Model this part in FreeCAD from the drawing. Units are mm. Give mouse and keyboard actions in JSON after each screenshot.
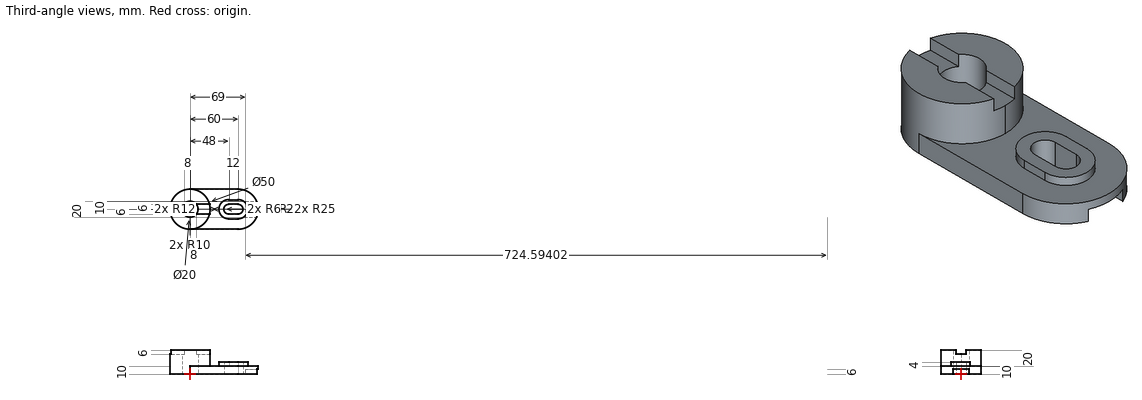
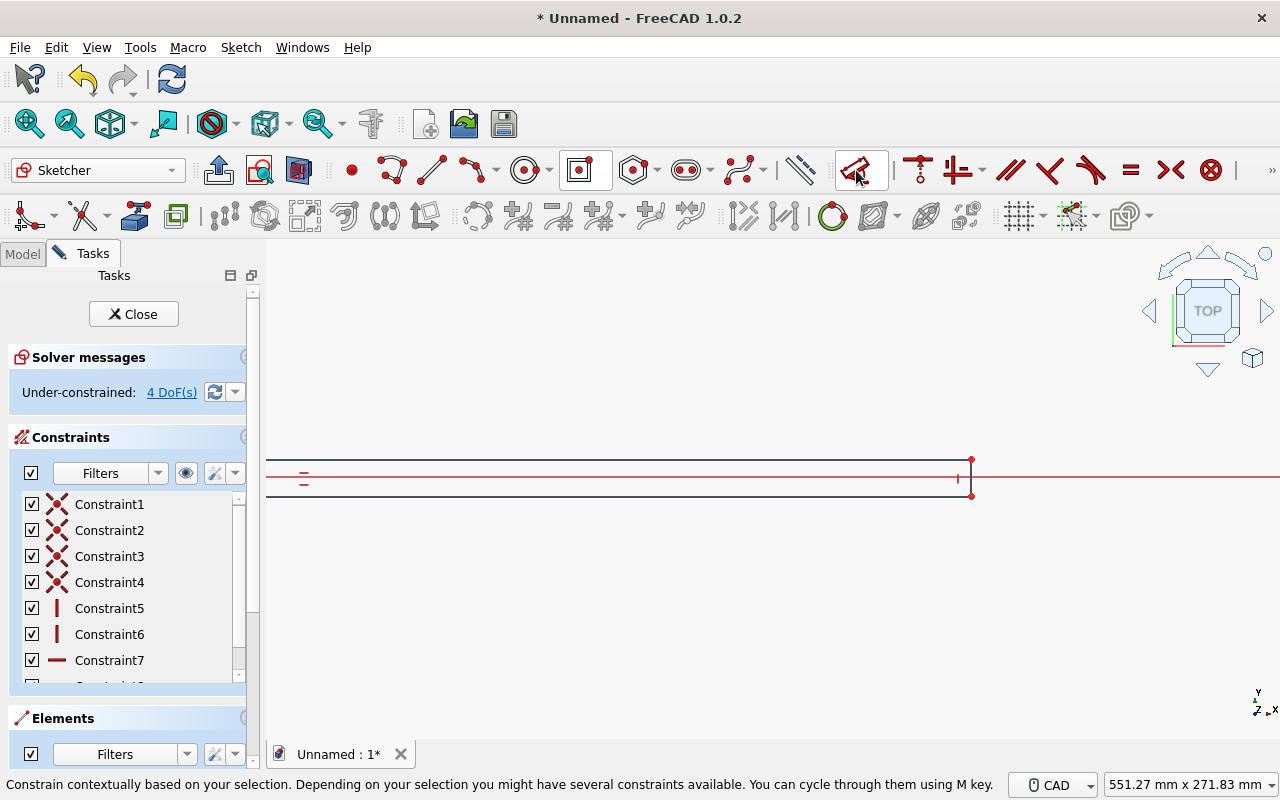
{"action": "scroll", "coordinate": [974, 496], "scroll_direction": "down", "scroll_amount": 5}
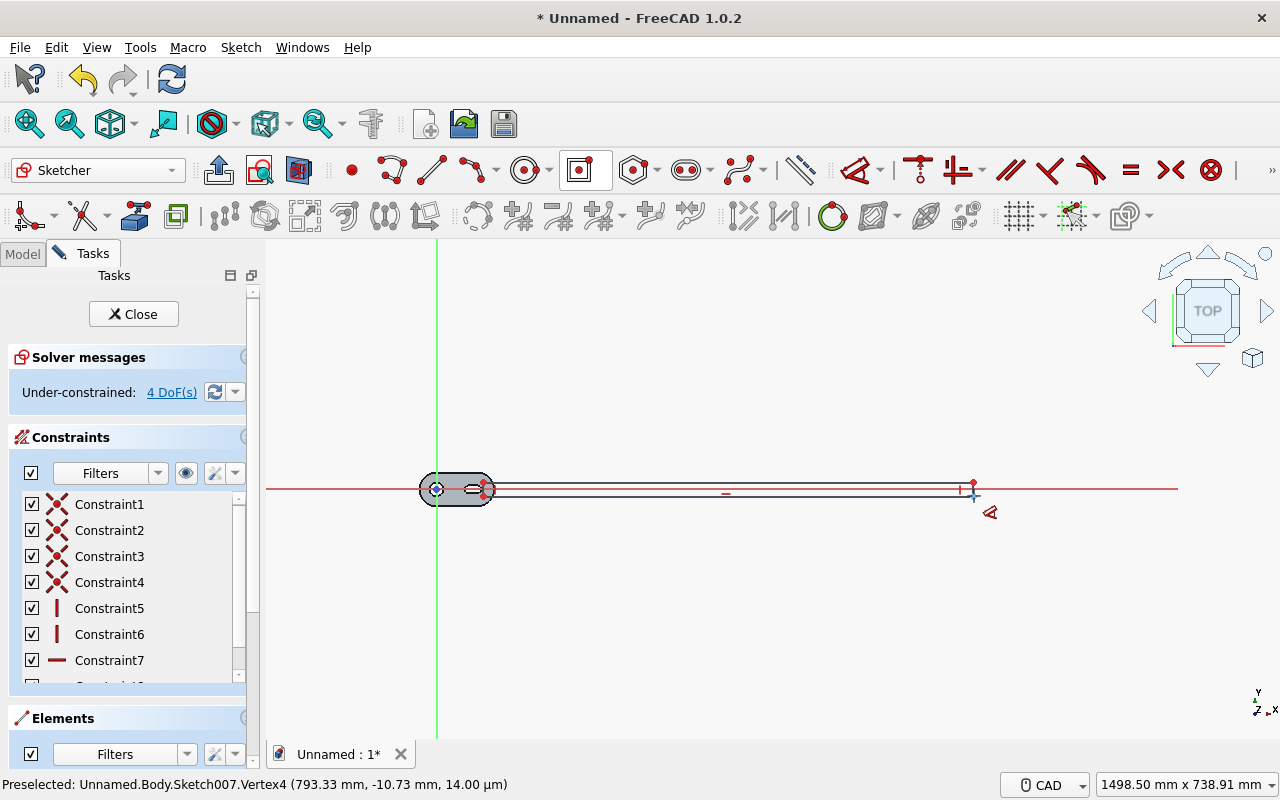
{"action": "scroll", "coordinate": [483, 488], "scroll_direction": "up", "scroll_amount": 6}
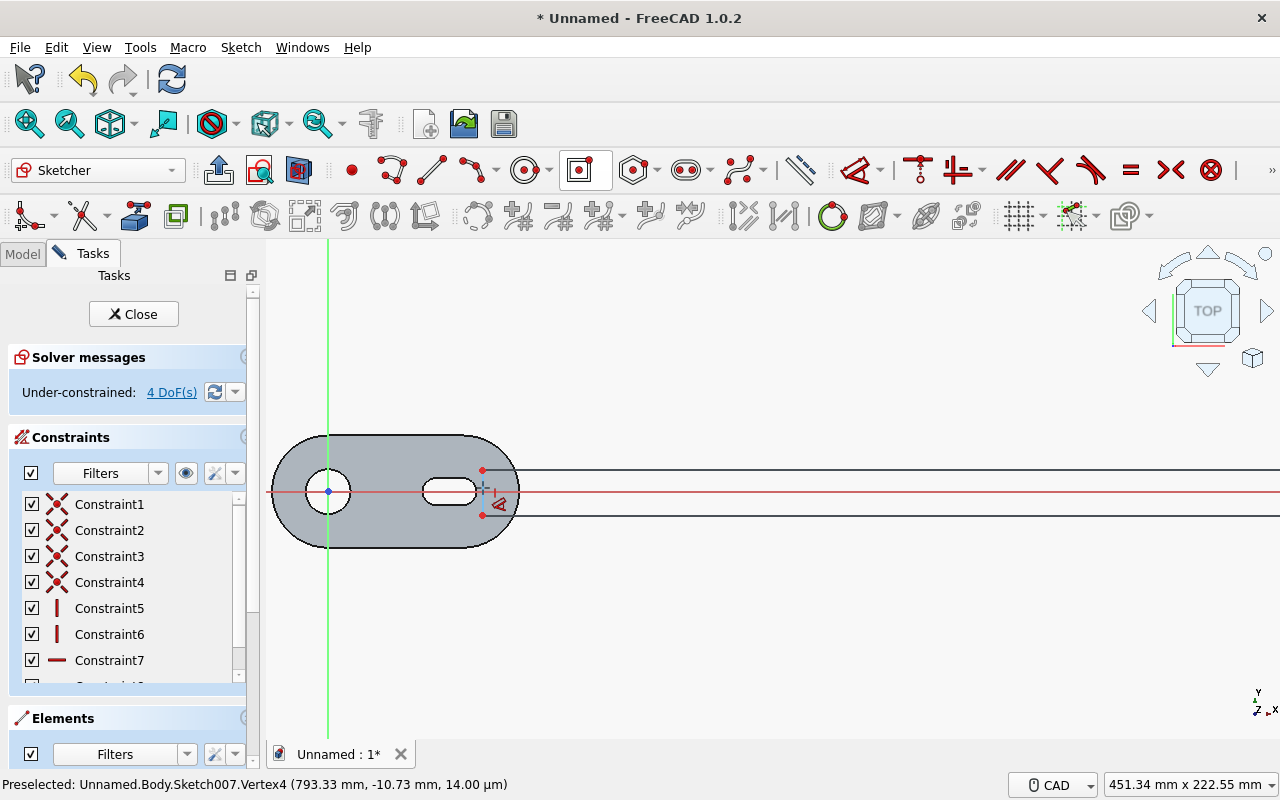
{"action": "left_click", "coordinate": [483, 488]}
{"action": "left_click", "coordinate": [449, 477]}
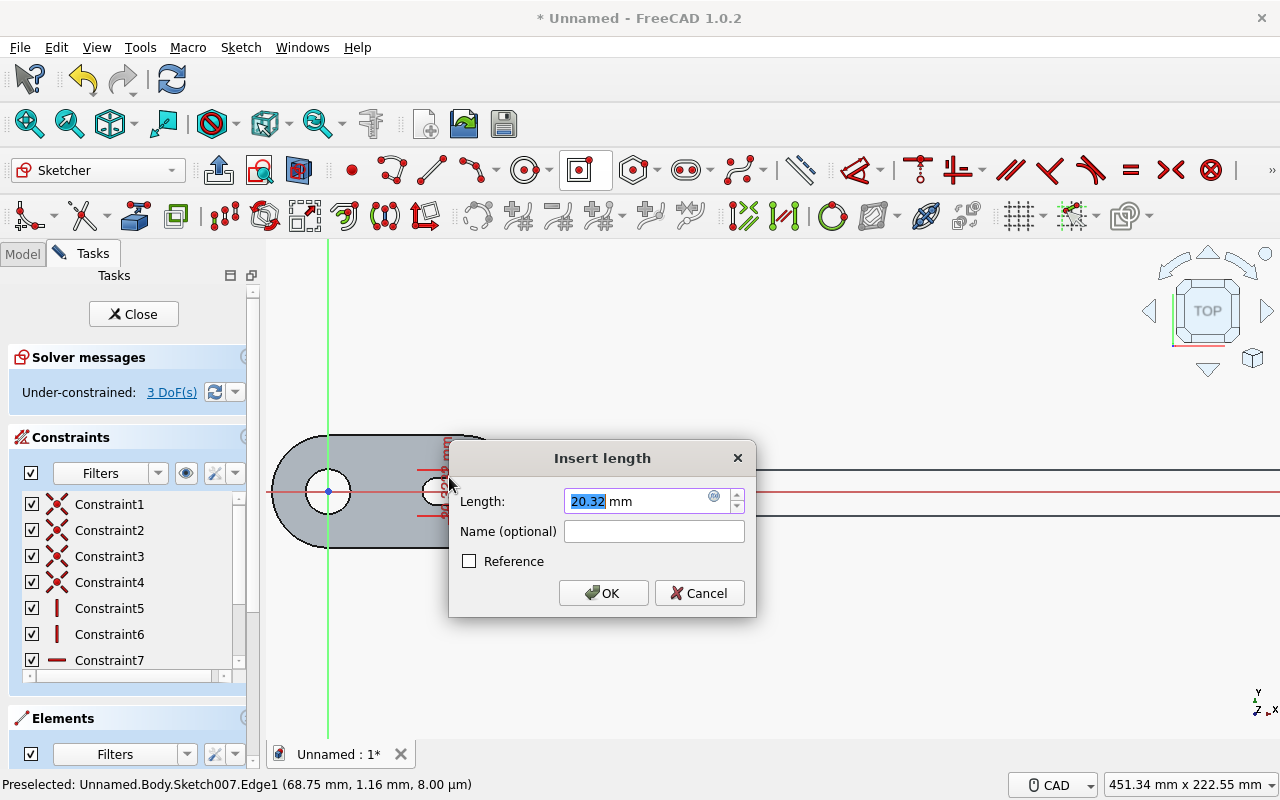
{"action": "type", "text": "20"}
{"action": "key", "text": "Return"}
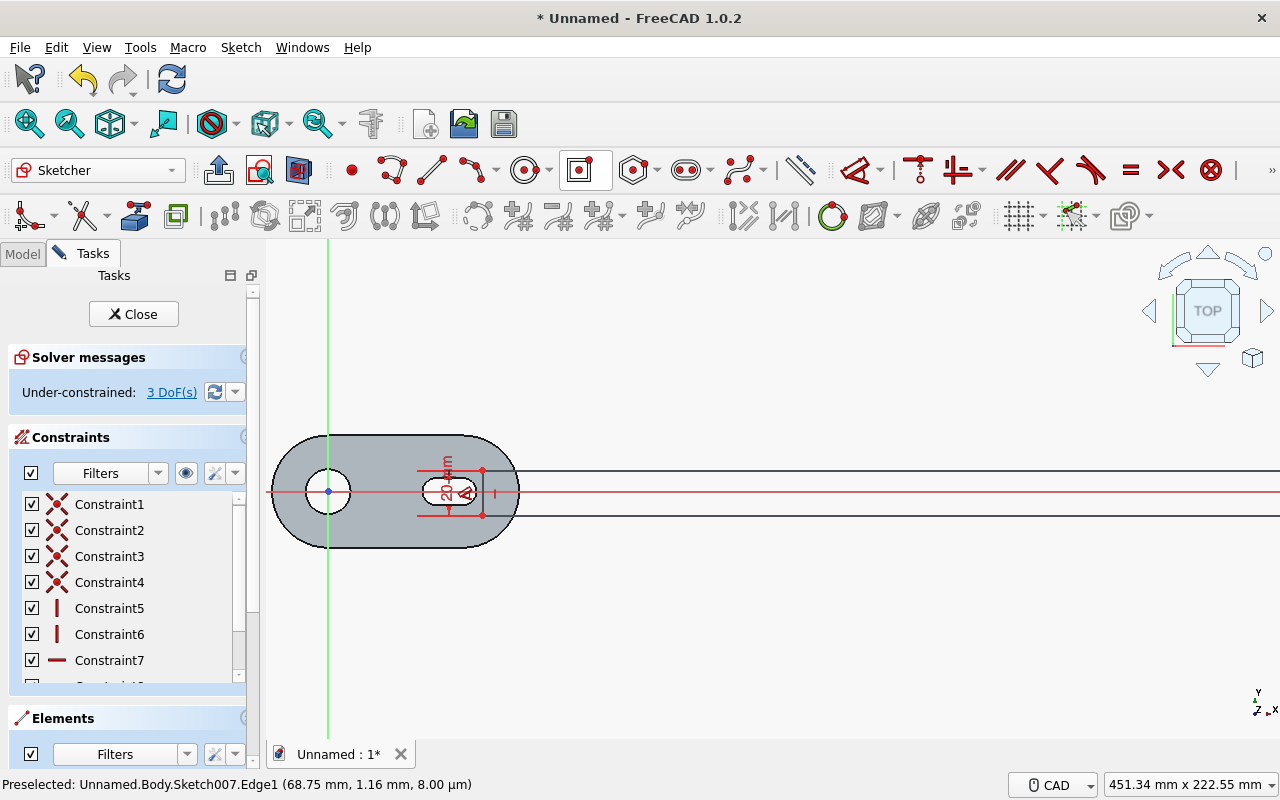
{"action": "left_click", "coordinate": [483, 471]}
{"action": "left_click", "coordinate": [405, 437]}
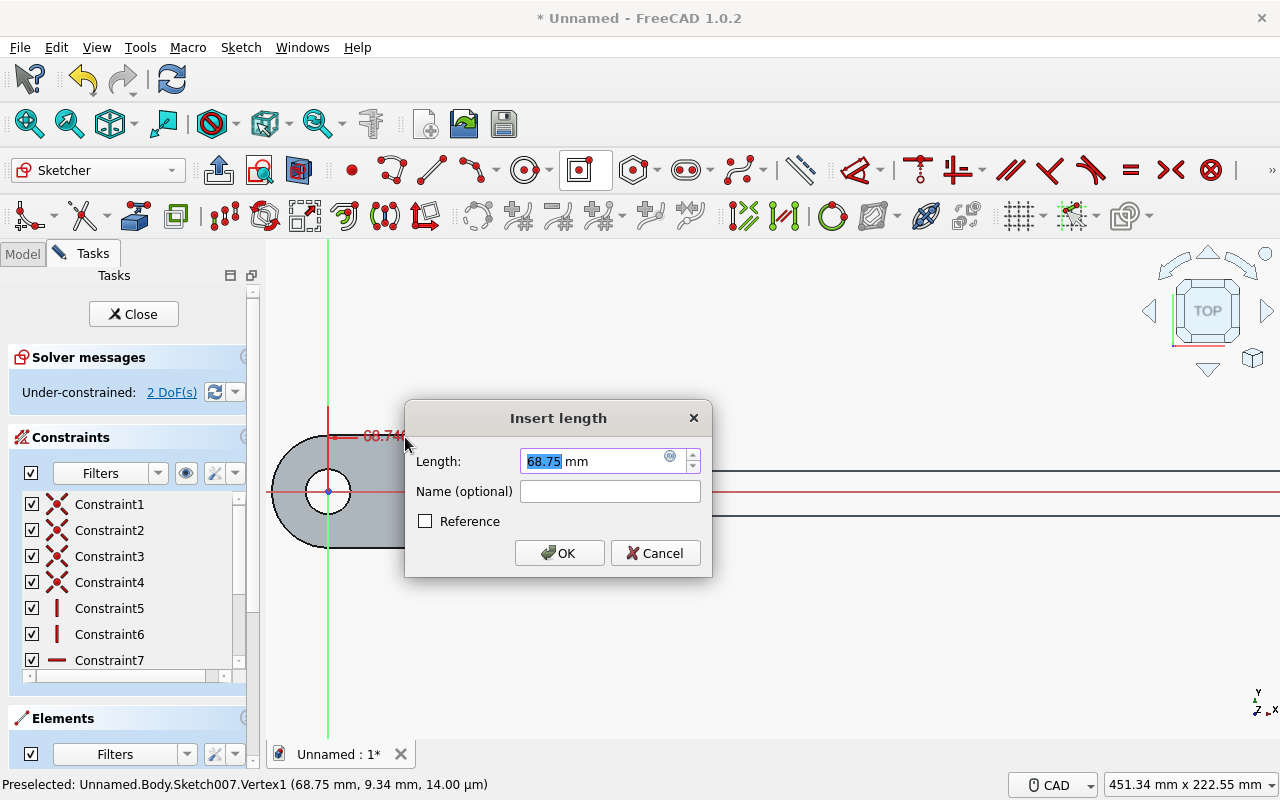
{"action": "type", "text": "69"}
{"action": "key", "text": "Return"}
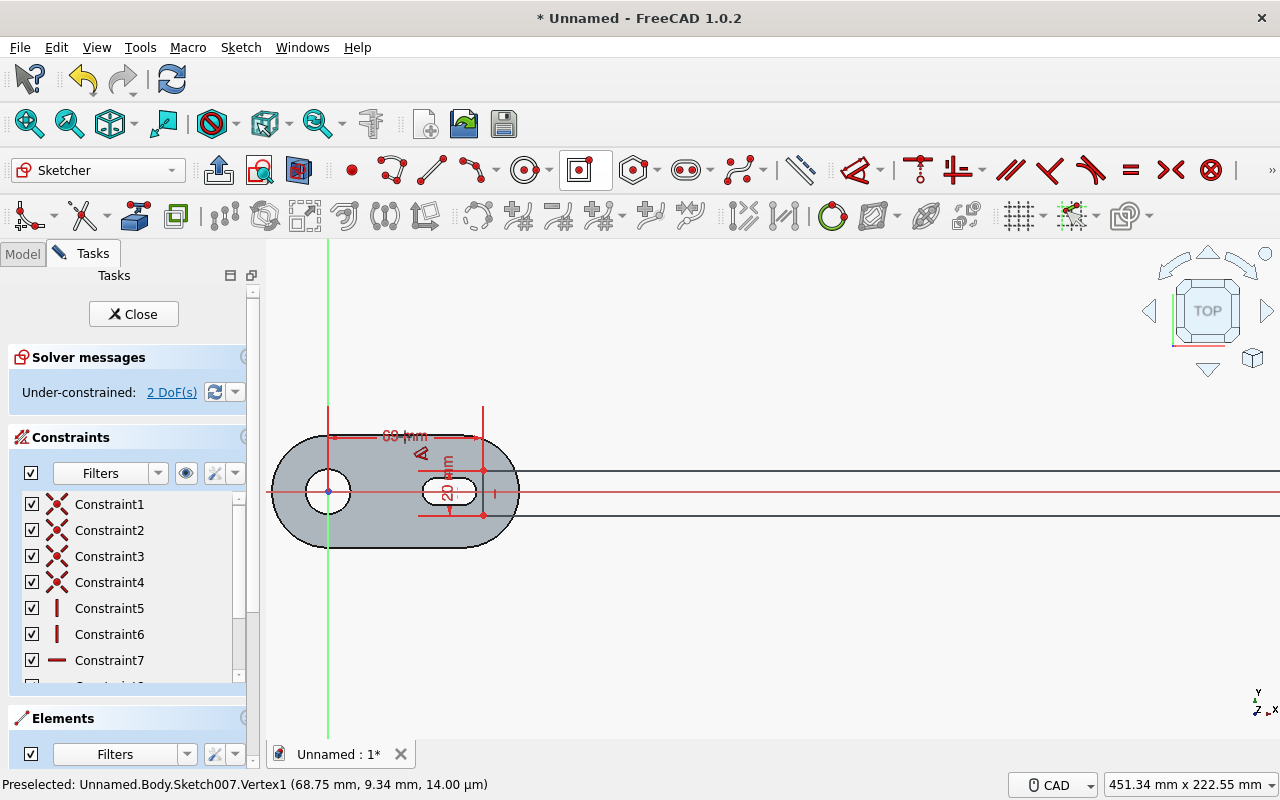
{"action": "scroll", "coordinate": [483, 471], "scroll_direction": "up", "scroll_amount": 3}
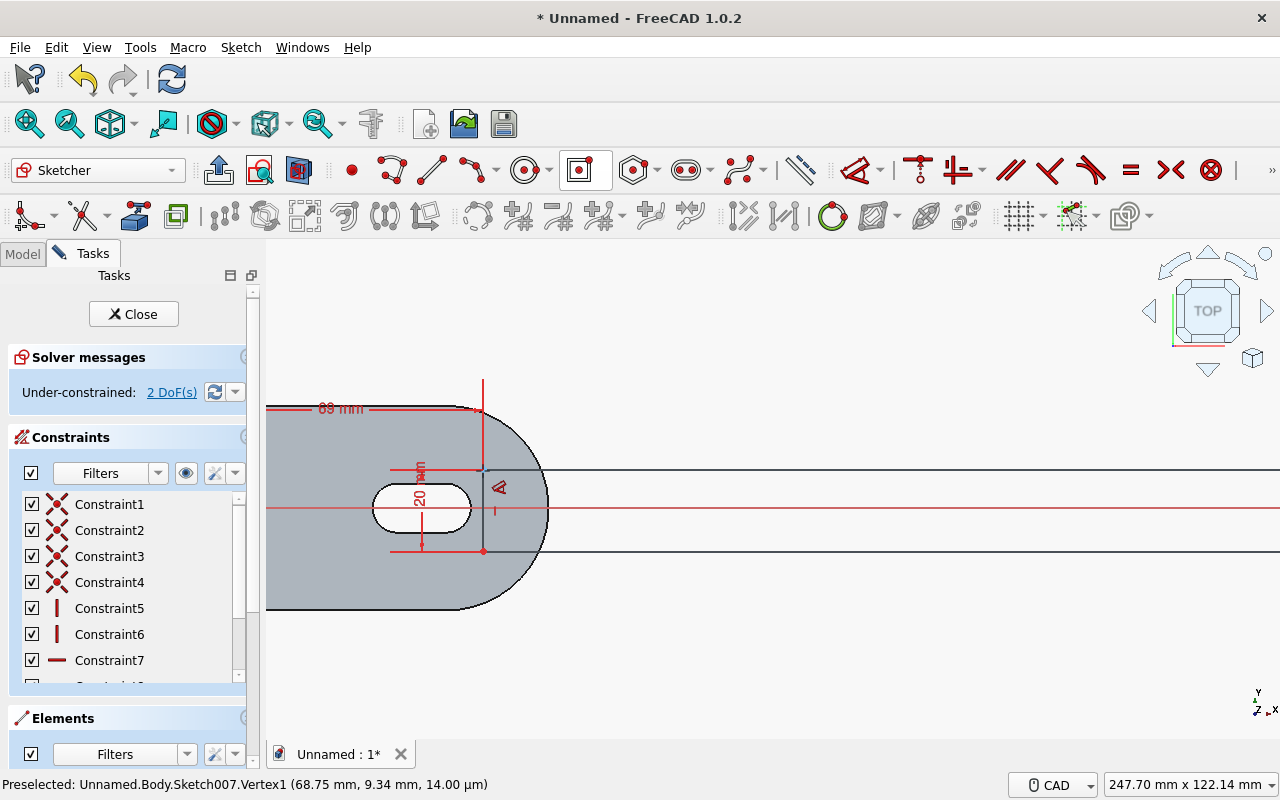
{"action": "left_click", "coordinate": [483, 470]}
{"action": "left_click", "coordinate": [517, 489]}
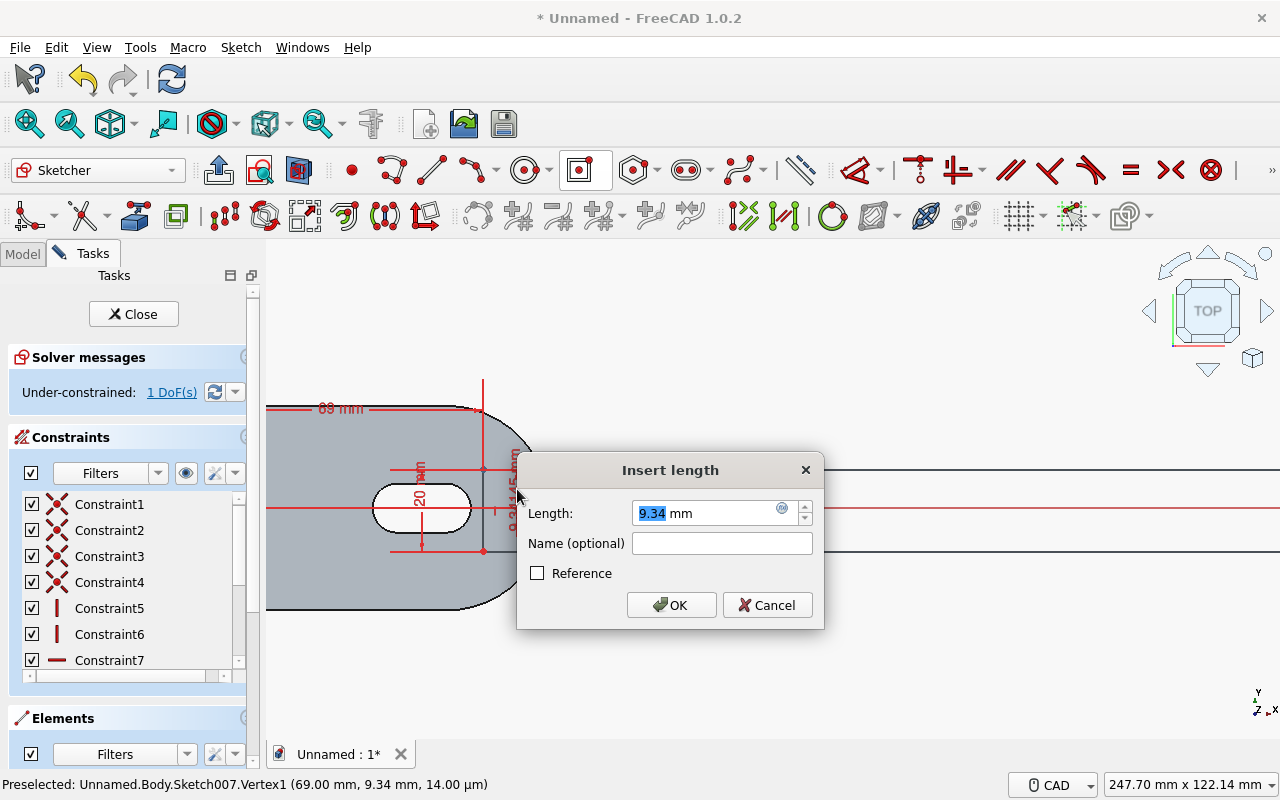
{"action": "type", "text": "10"}
{"action": "key", "text": "Return"}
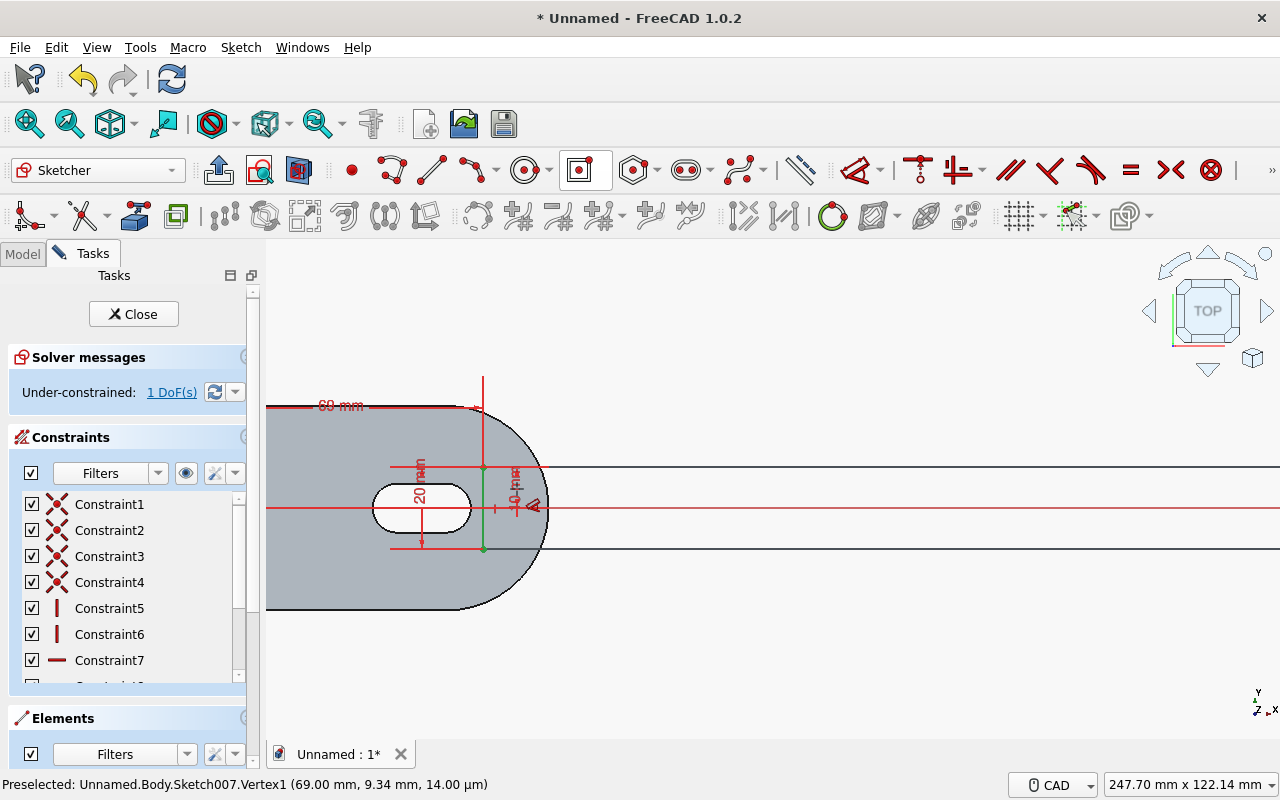
{"action": "scroll", "coordinate": [483, 485], "scroll_direction": "down", "scroll_amount": 9}